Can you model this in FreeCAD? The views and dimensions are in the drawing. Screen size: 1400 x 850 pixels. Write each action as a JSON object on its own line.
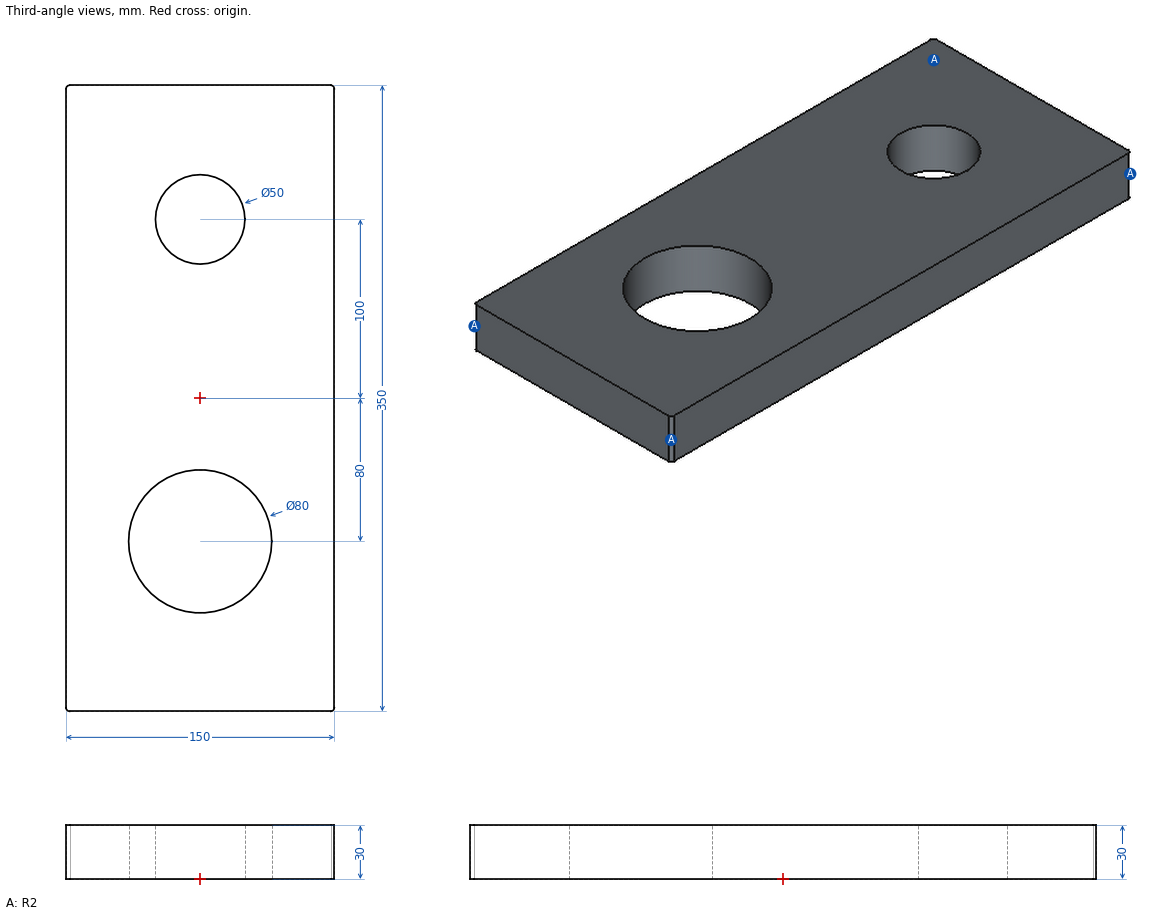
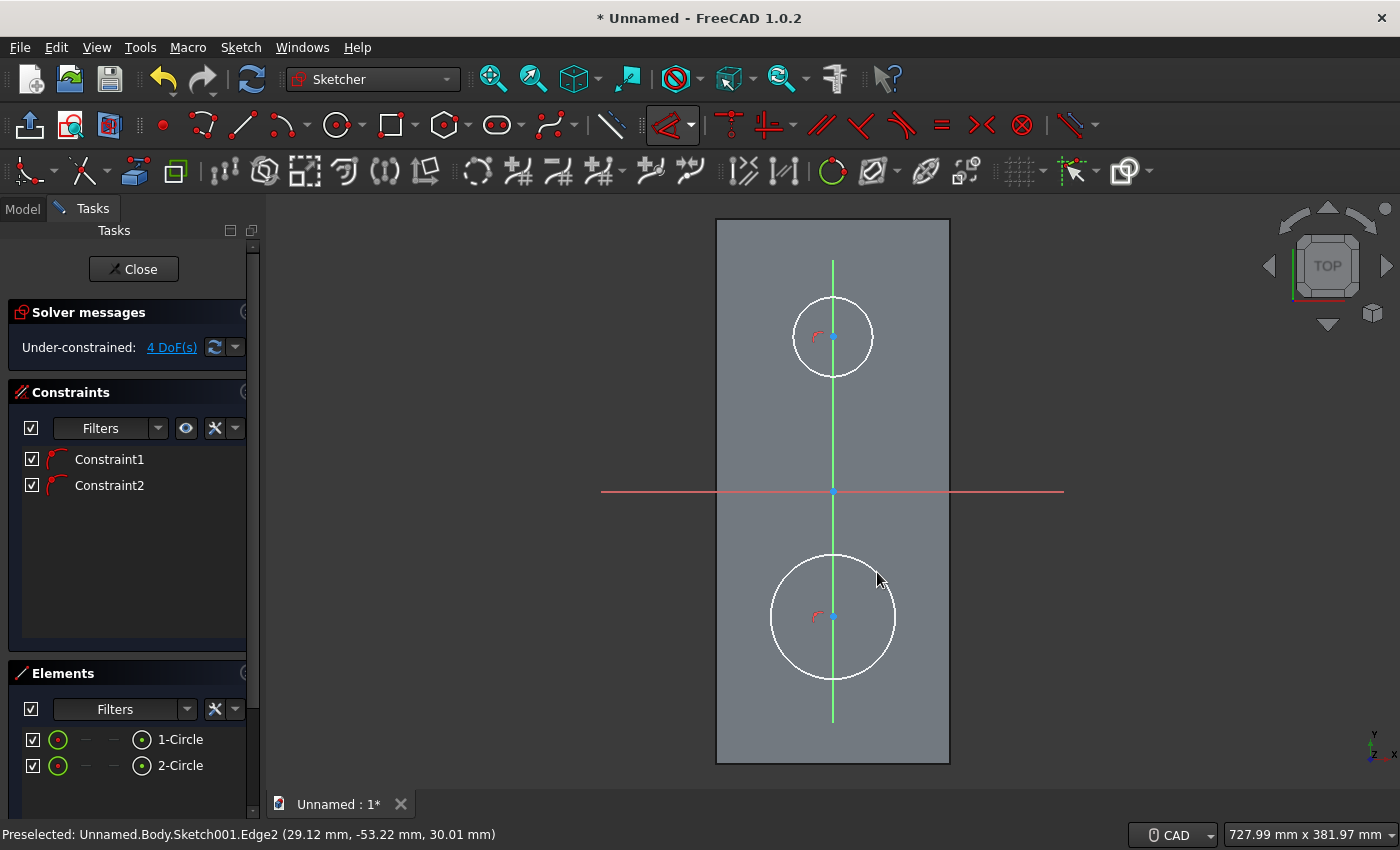
{"action": "left_click", "coordinate": [861, 309]}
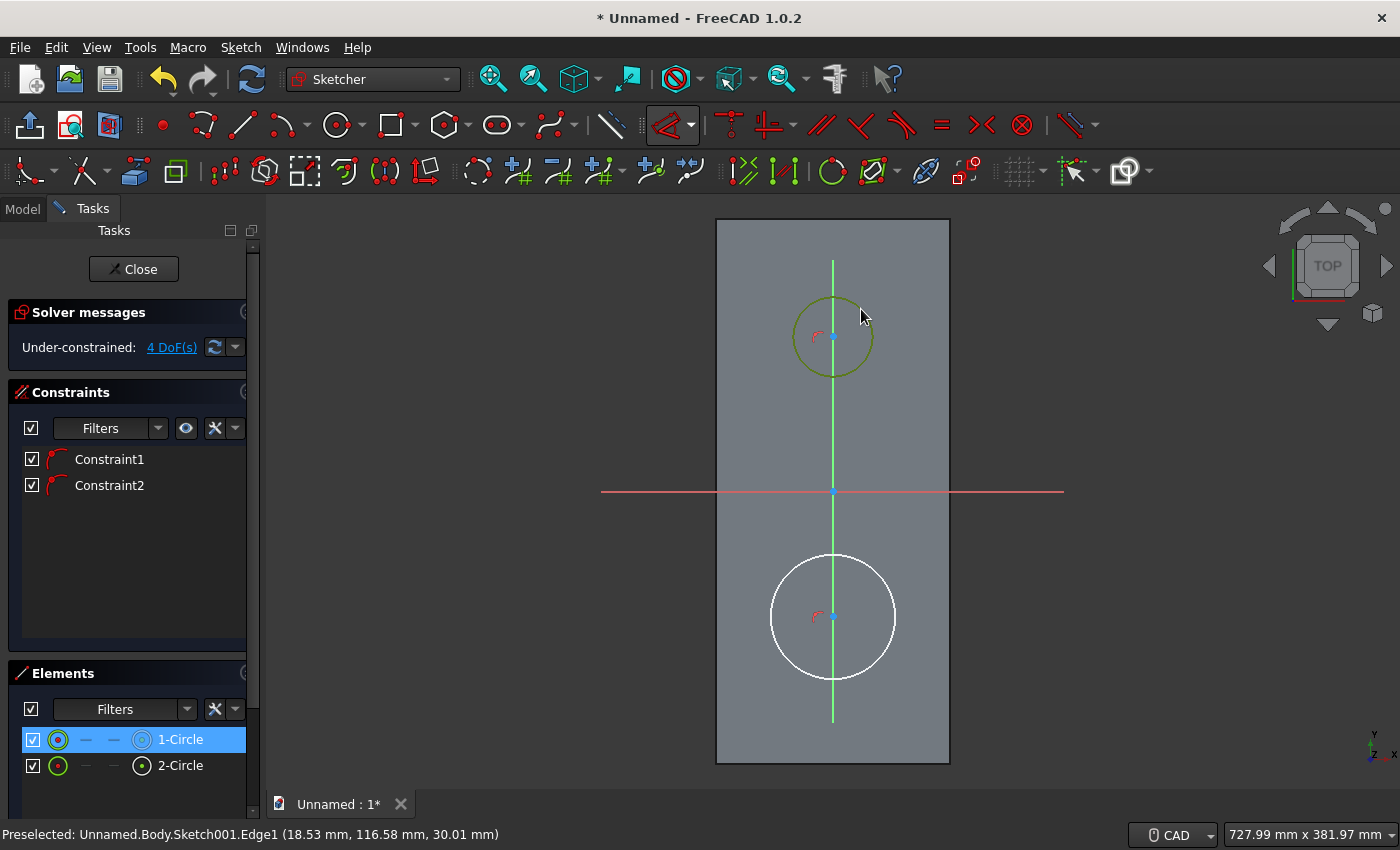
{"action": "key", "text": "k o"}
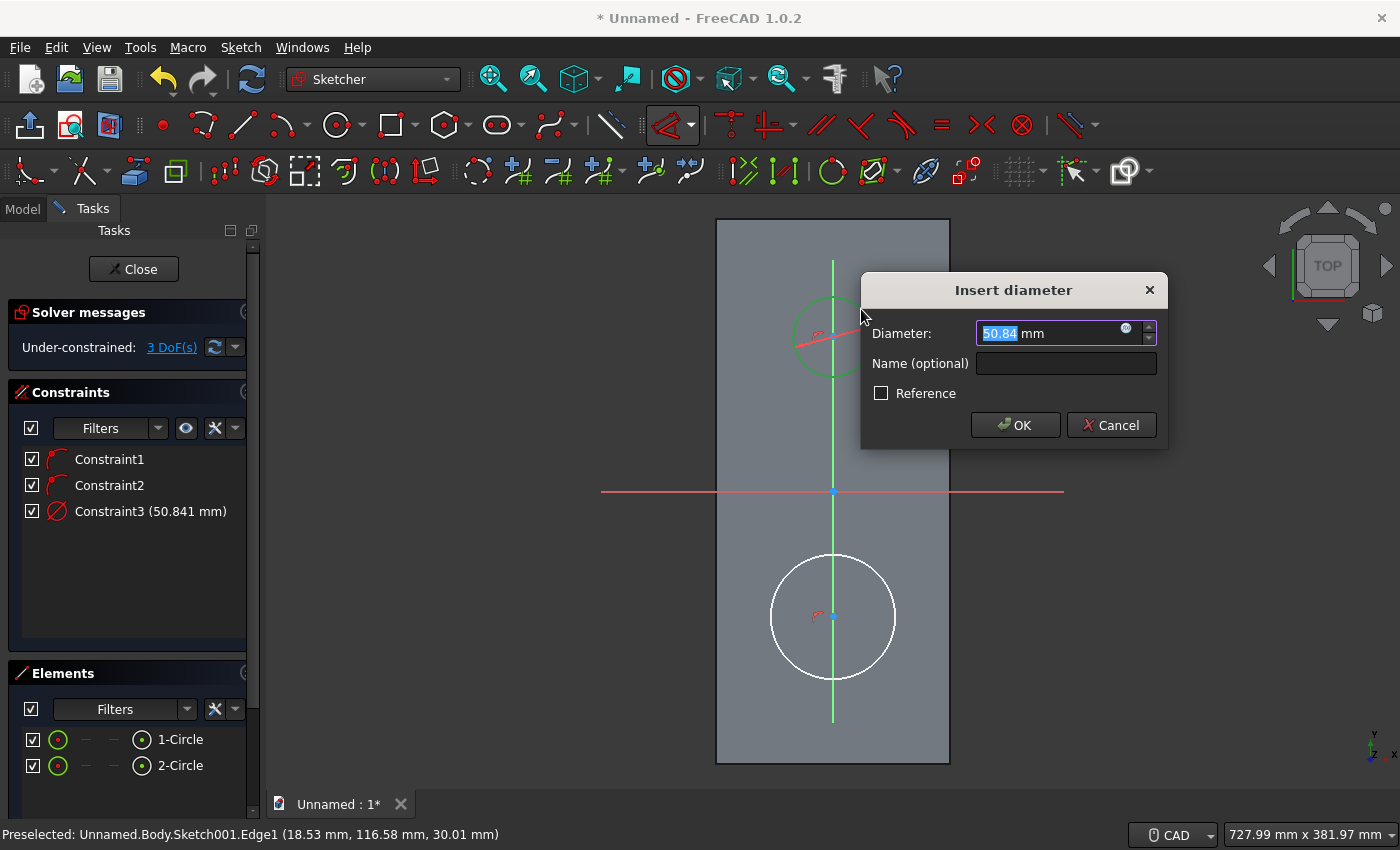
{"action": "type", "text": "50"}
{"action": "key", "text": "Return"}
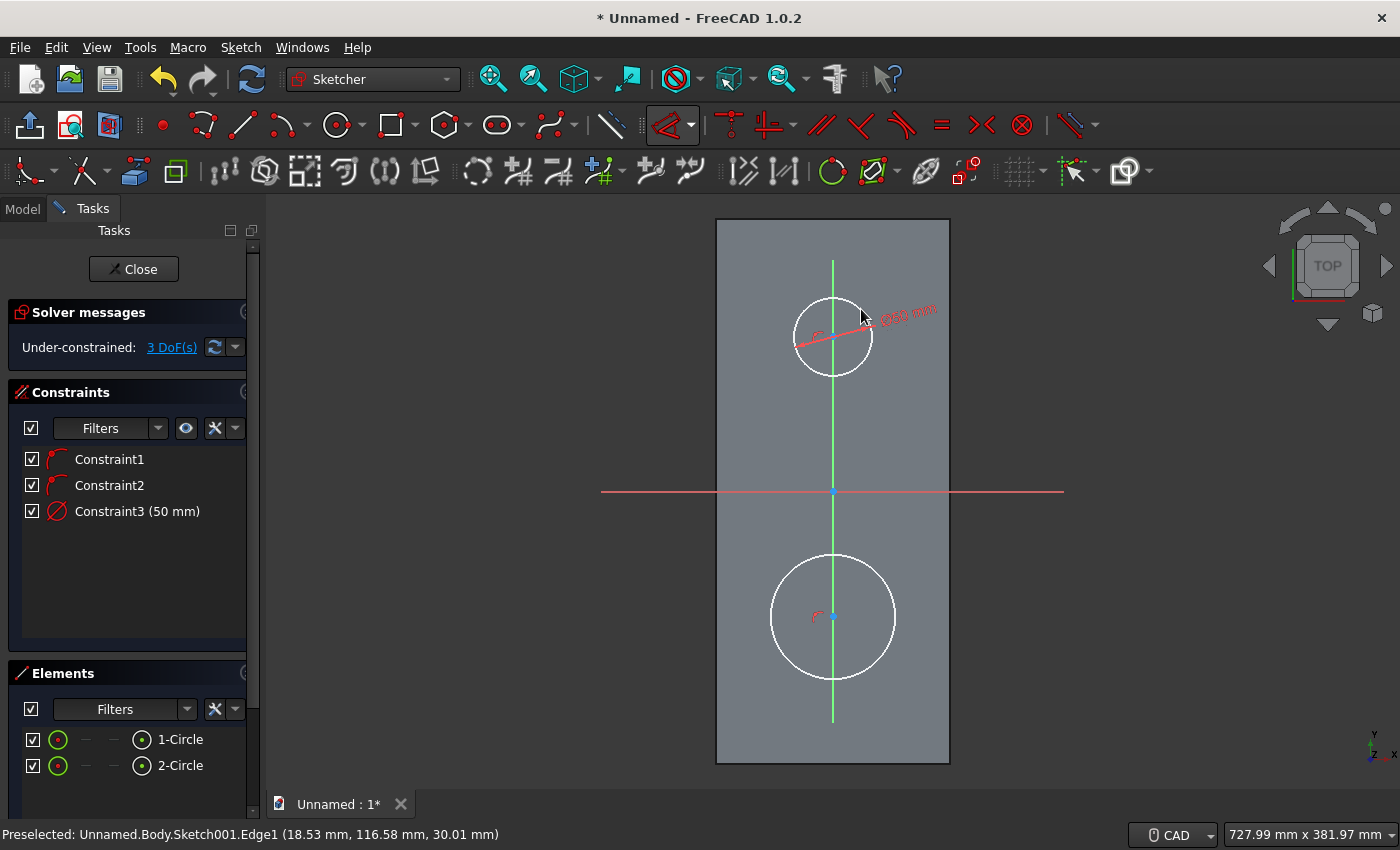
{"action": "left_click", "coordinate": [877, 573]}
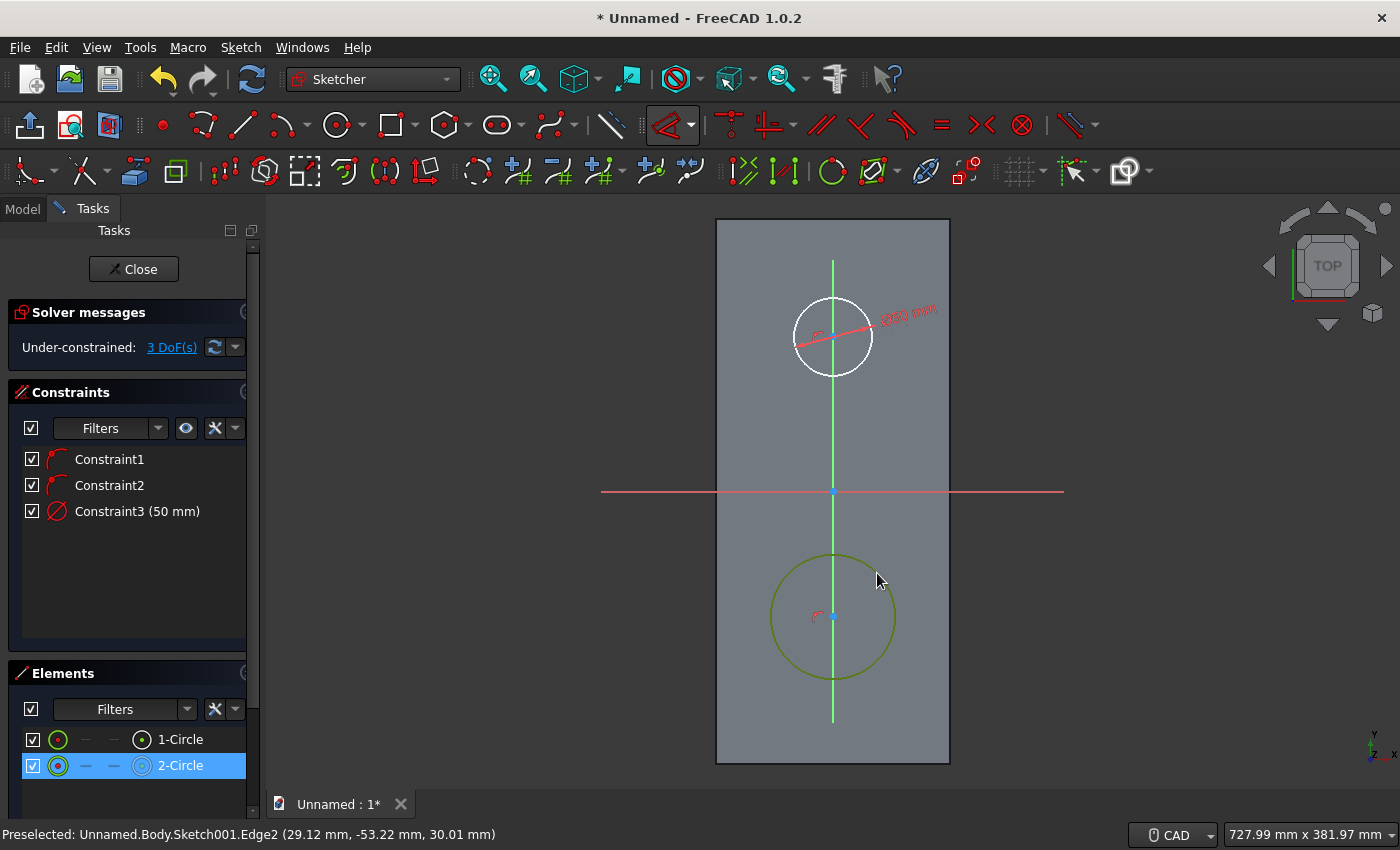
{"action": "key", "text": "k o"}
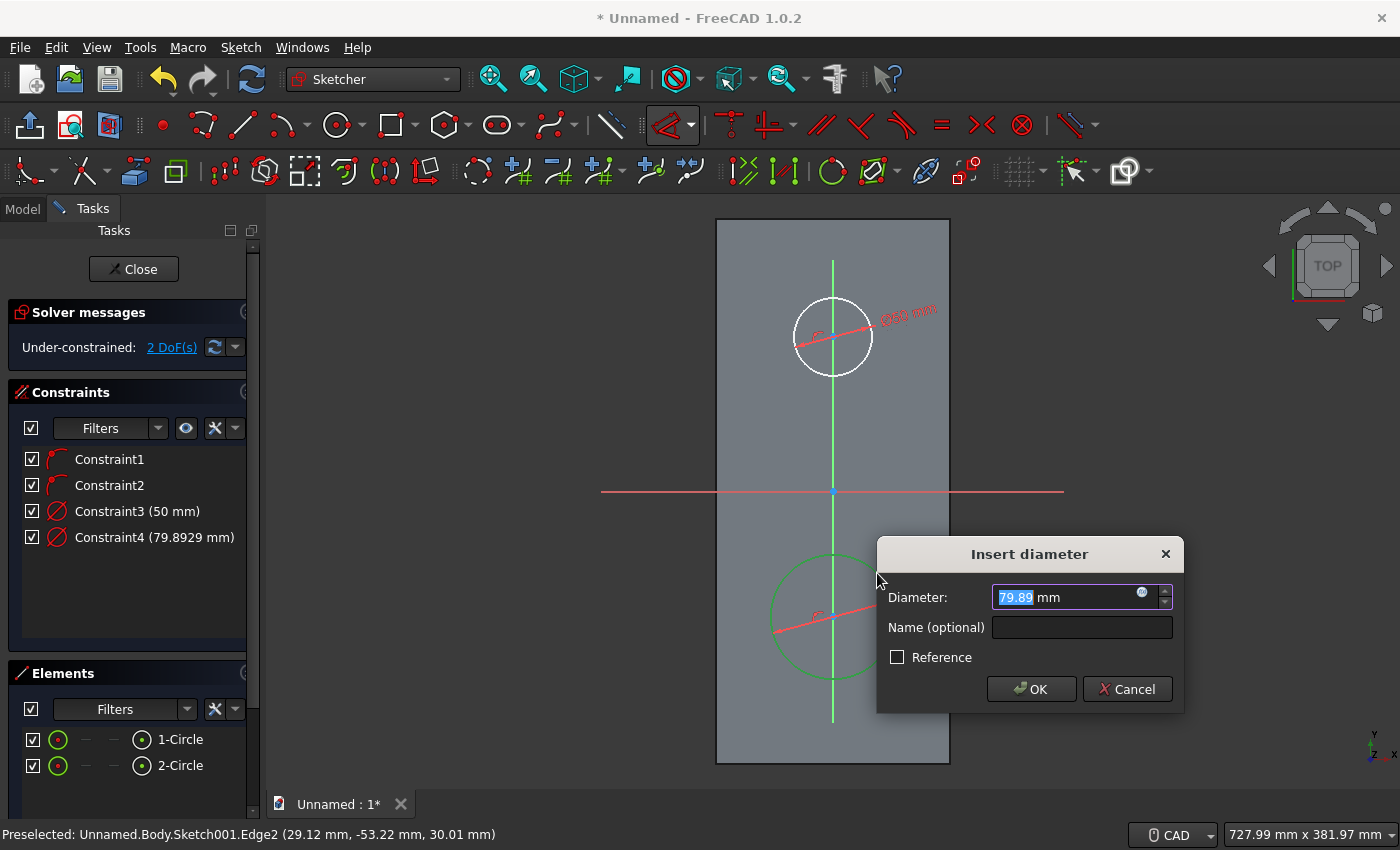
{"action": "type", "text": "80"}
{"action": "key", "text": "Return"}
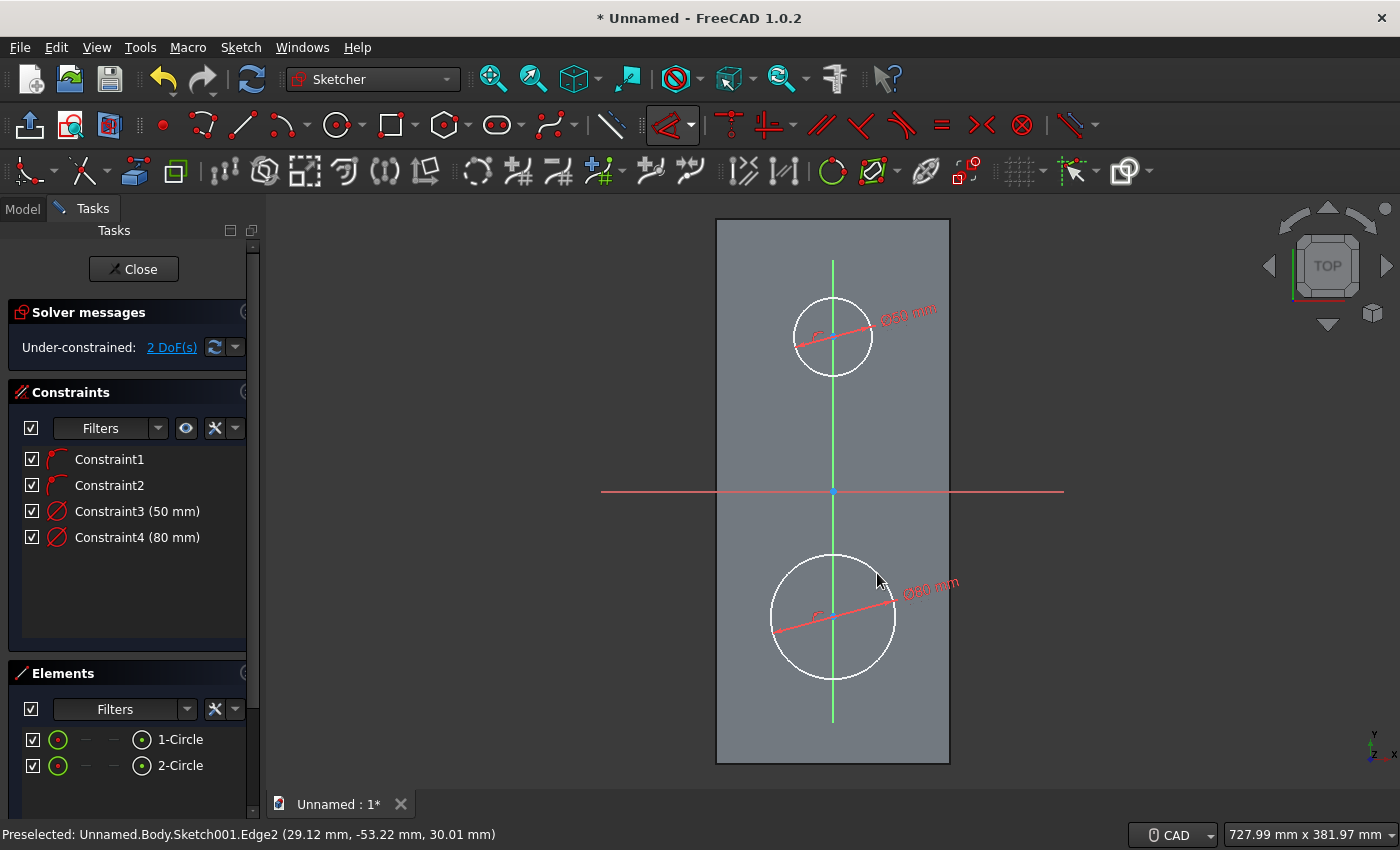
{"action": "left_click", "coordinate": [833, 617]}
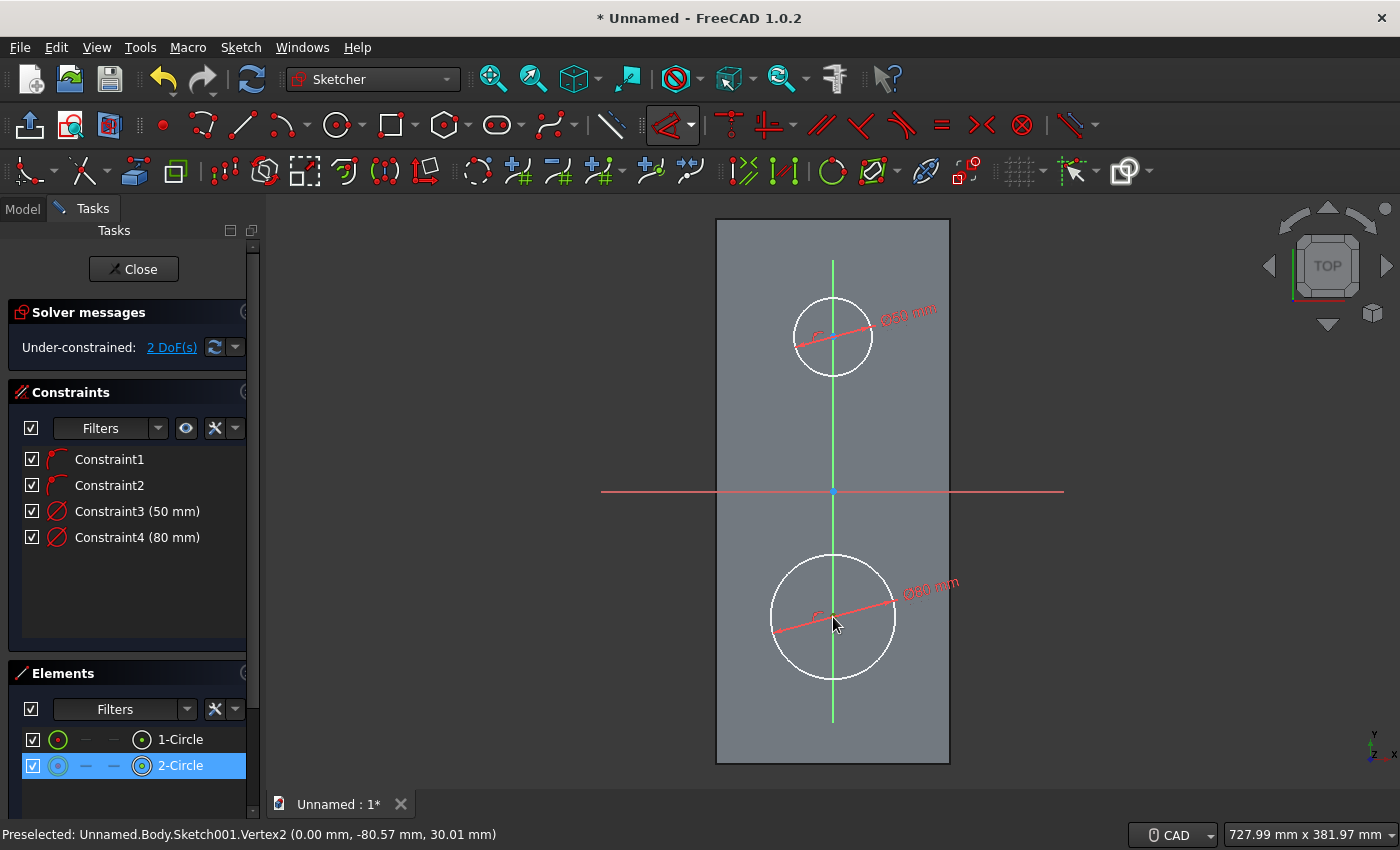
{"action": "left_click", "coordinate": [694, 126]}